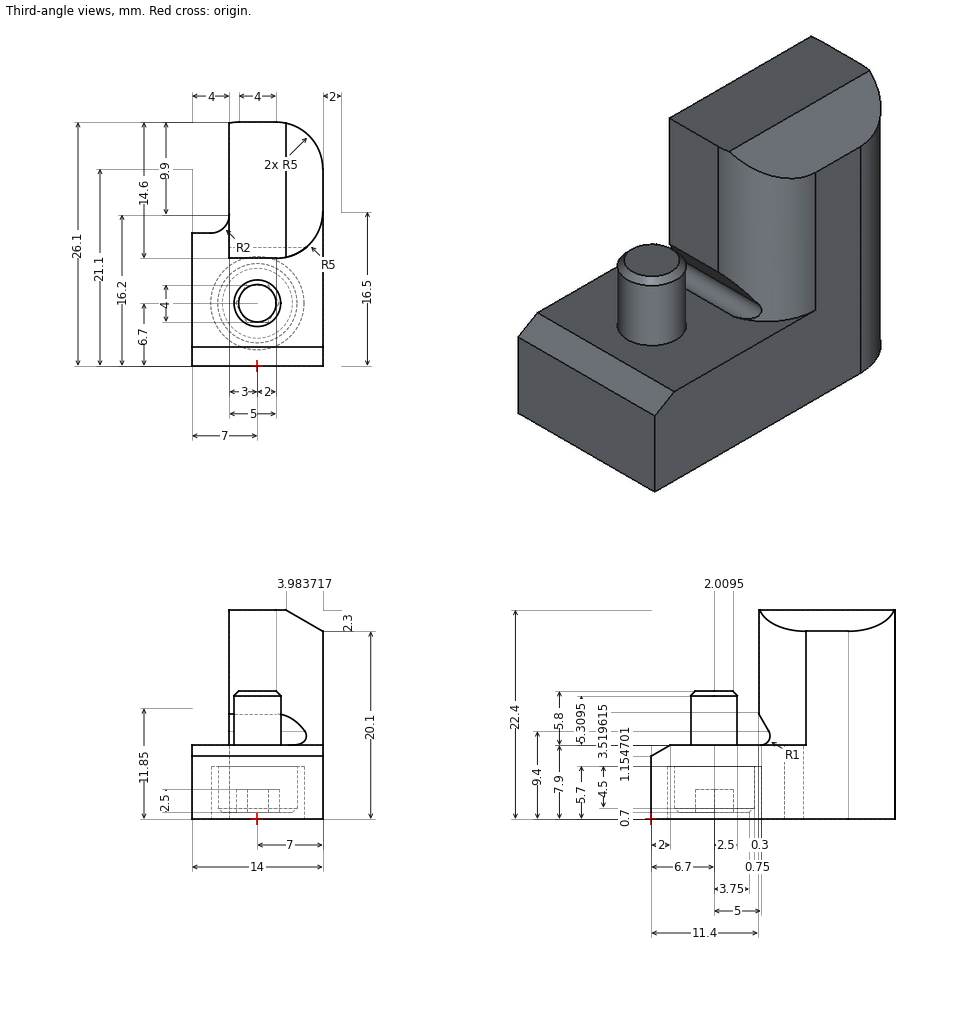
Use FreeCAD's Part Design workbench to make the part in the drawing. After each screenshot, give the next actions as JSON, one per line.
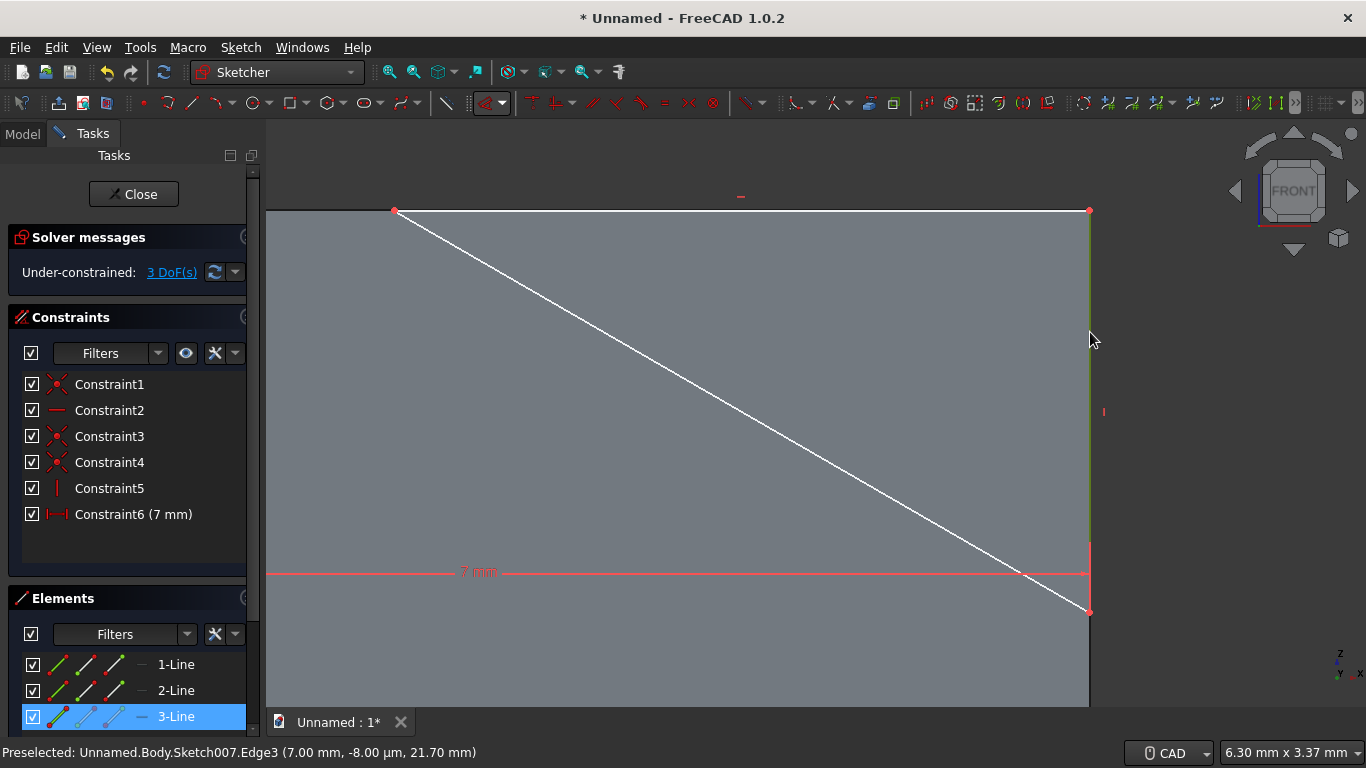
{"action": "key", "text": "i"}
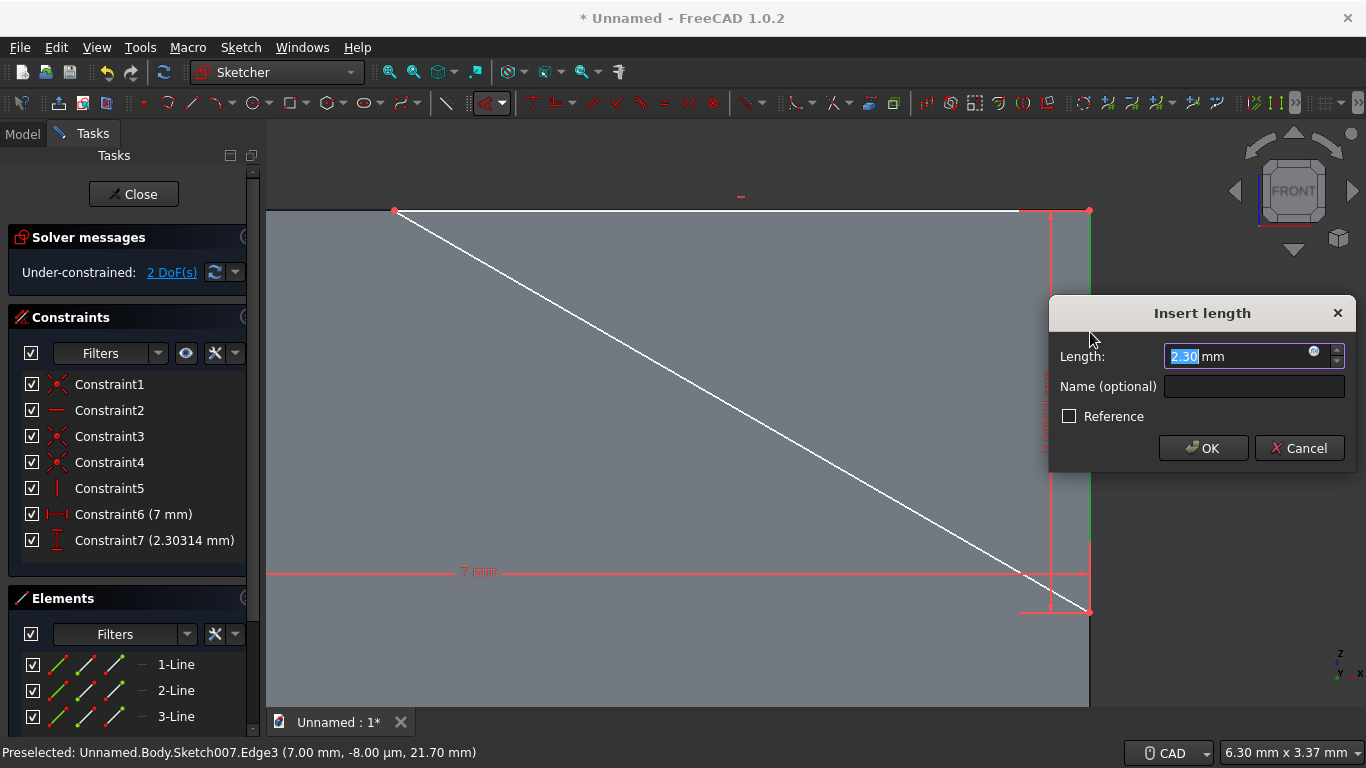
{"action": "type", "text": "2.3"}
{"action": "key", "text": "Return"}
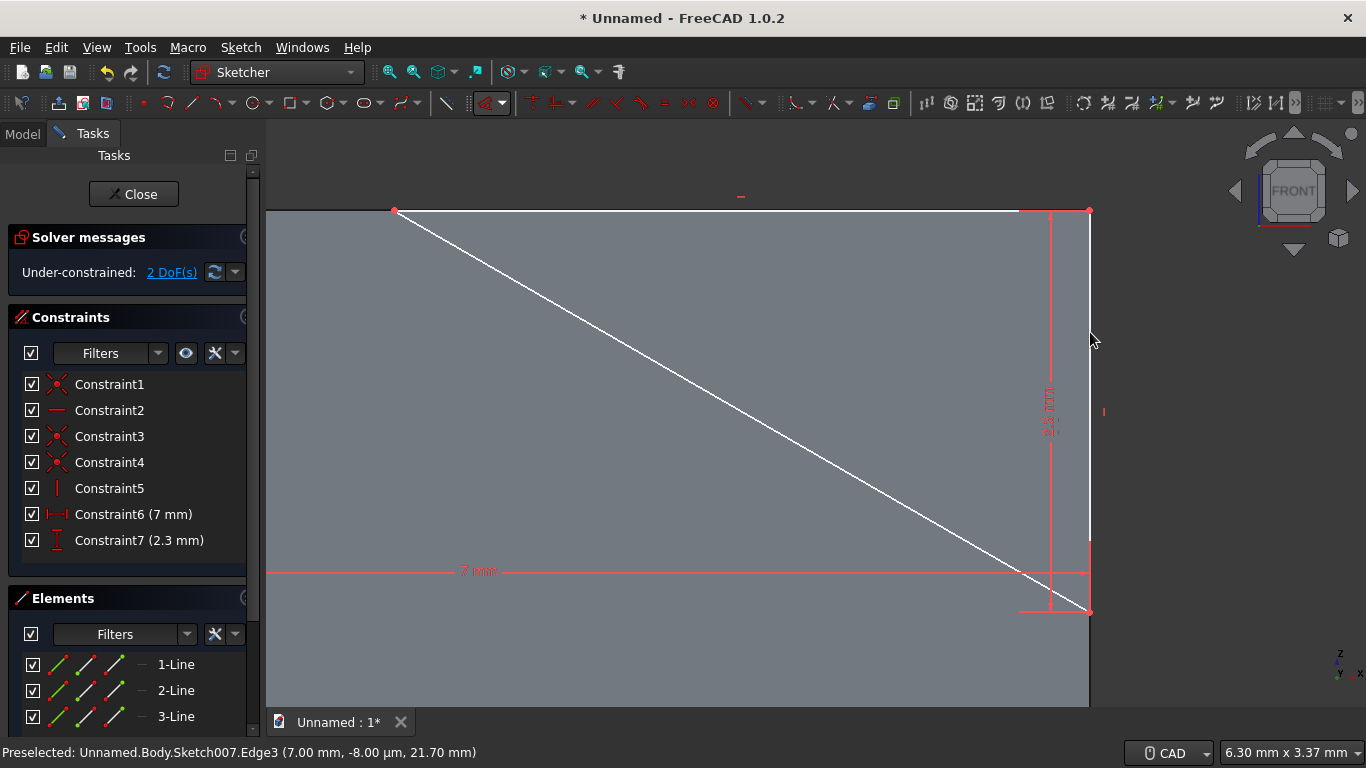
{"action": "left_click", "coordinate": [1090, 612]}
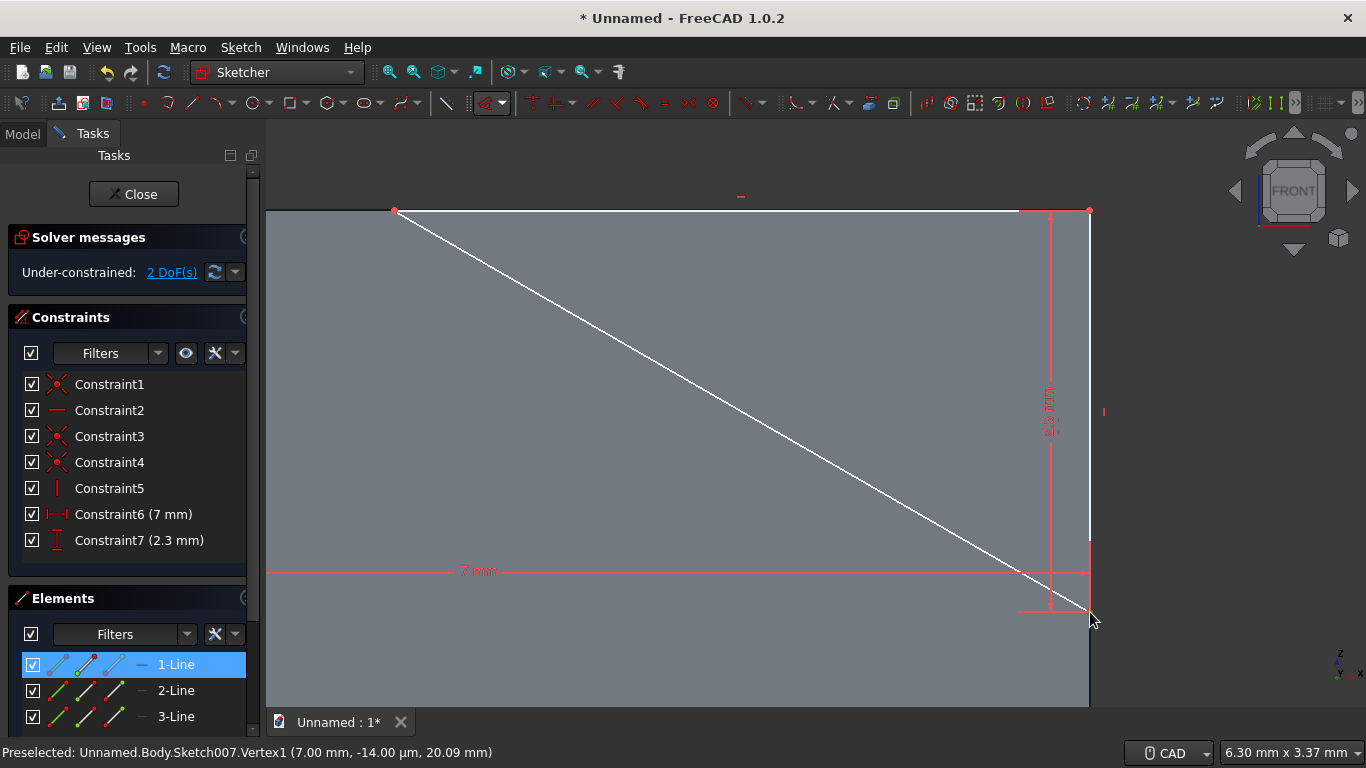
{"action": "left_click", "coordinate": [504, 104]}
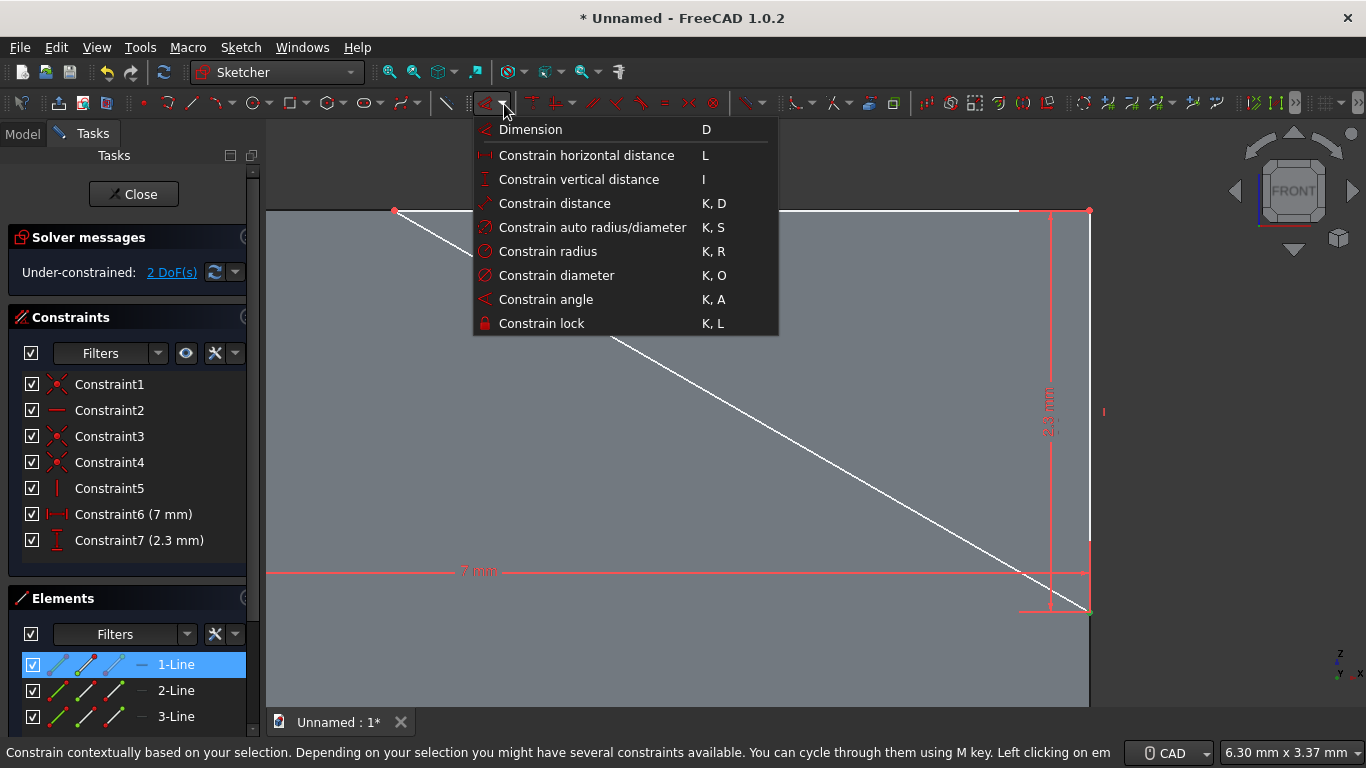
{"action": "left_click", "coordinate": [626, 179]}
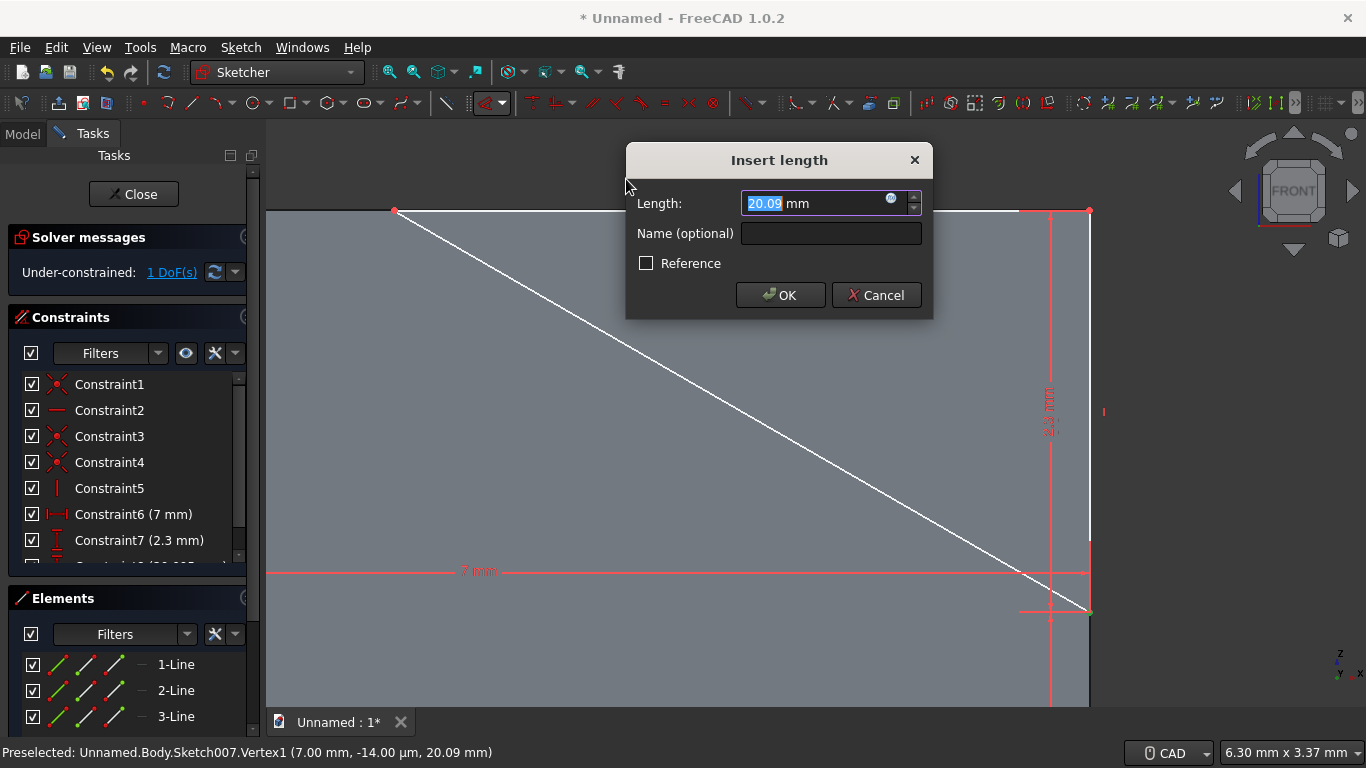
{"action": "type", "text": "20.1"}
{"action": "key", "text": "Return"}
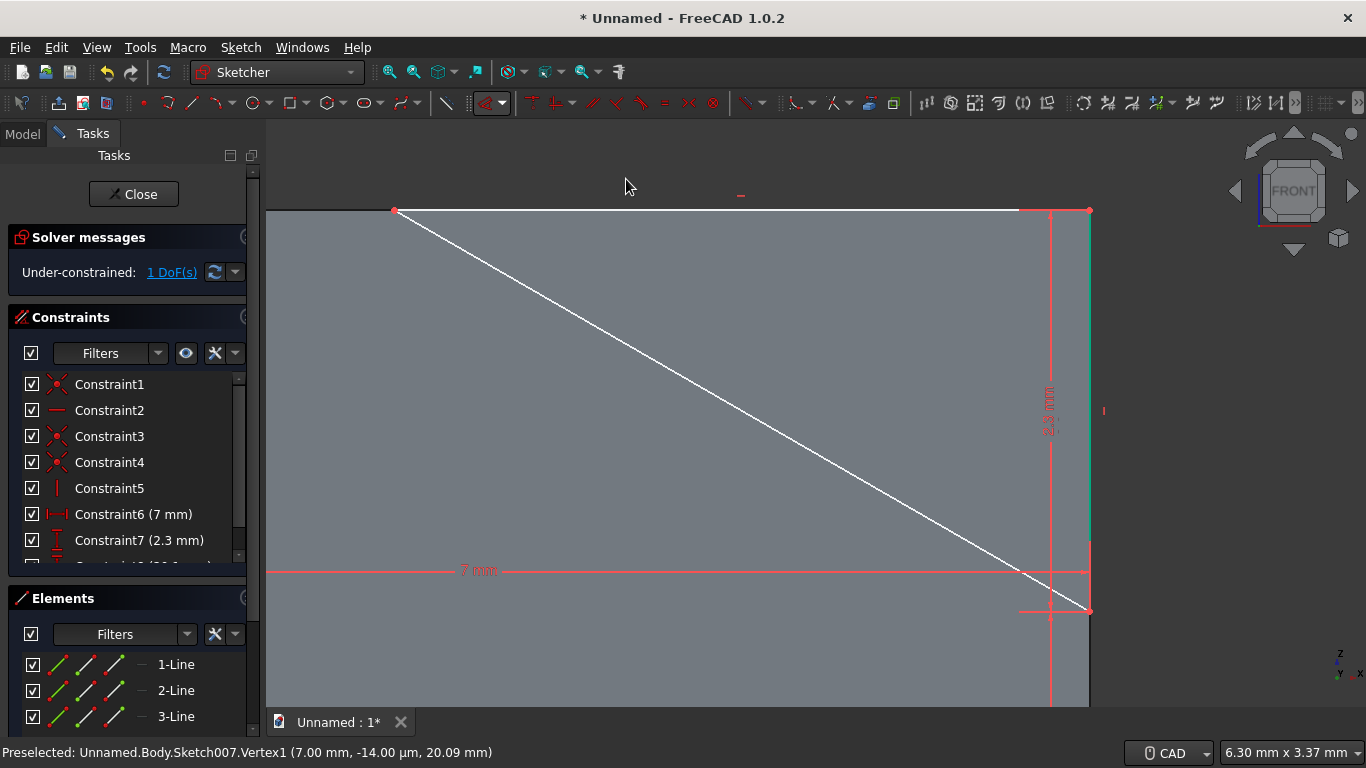
{"action": "left_click", "coordinate": [603, 210]}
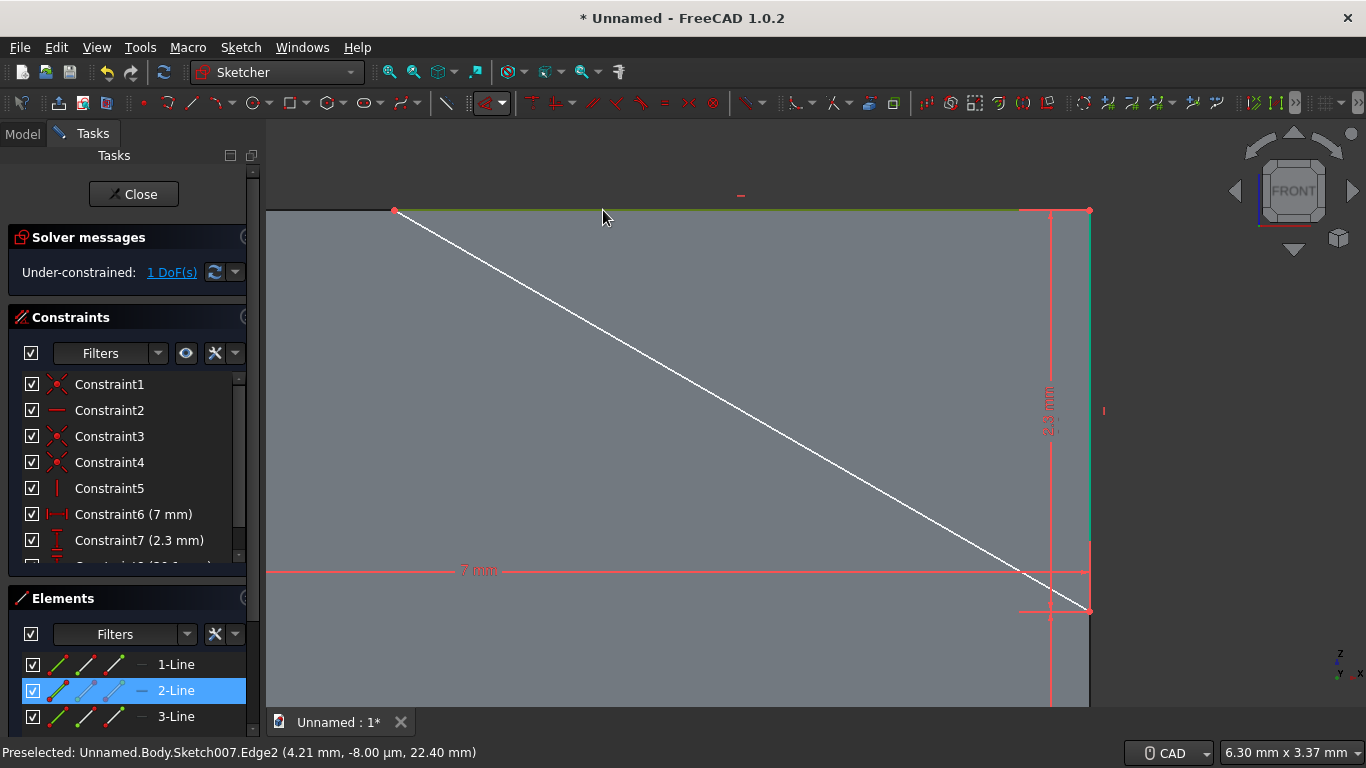
{"action": "key", "text": "l"}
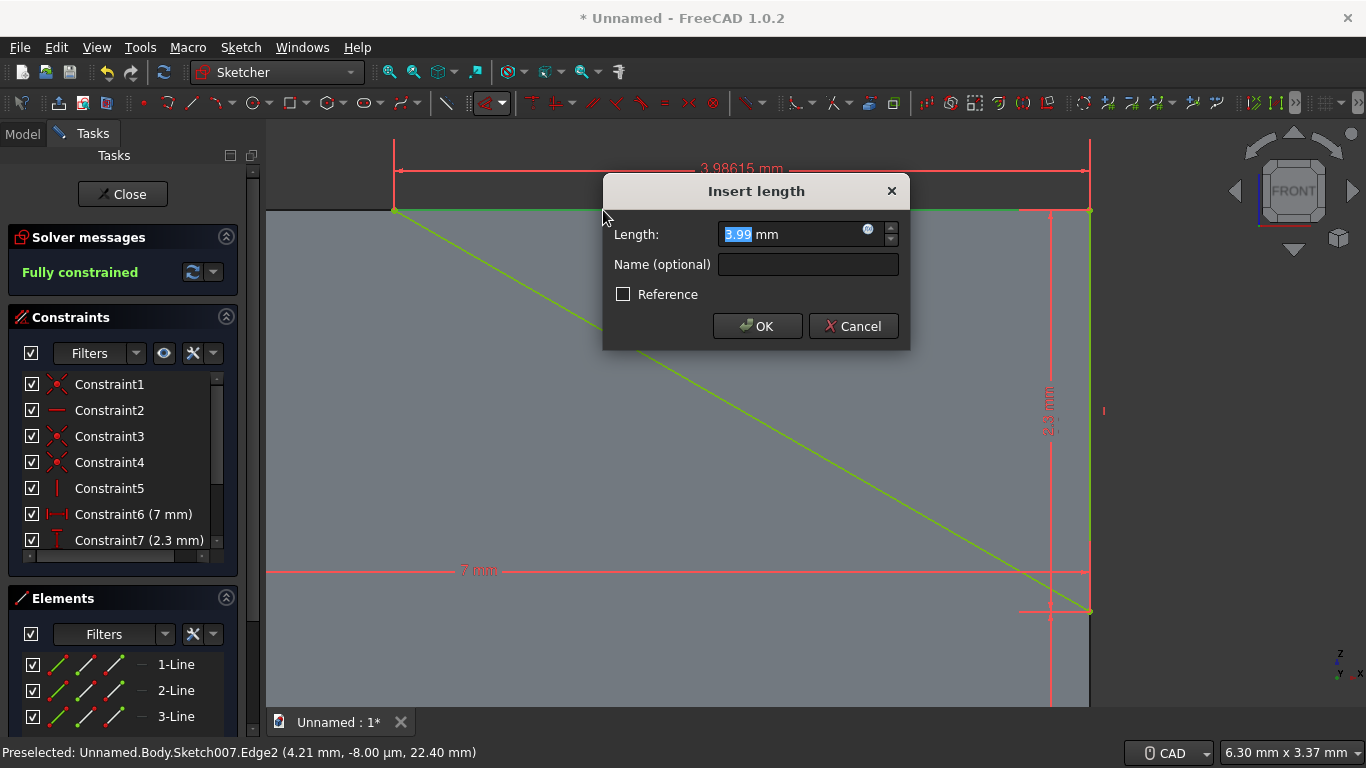
{"action": "type", "text": "3.983717"}
{"action": "key", "text": "Return"}